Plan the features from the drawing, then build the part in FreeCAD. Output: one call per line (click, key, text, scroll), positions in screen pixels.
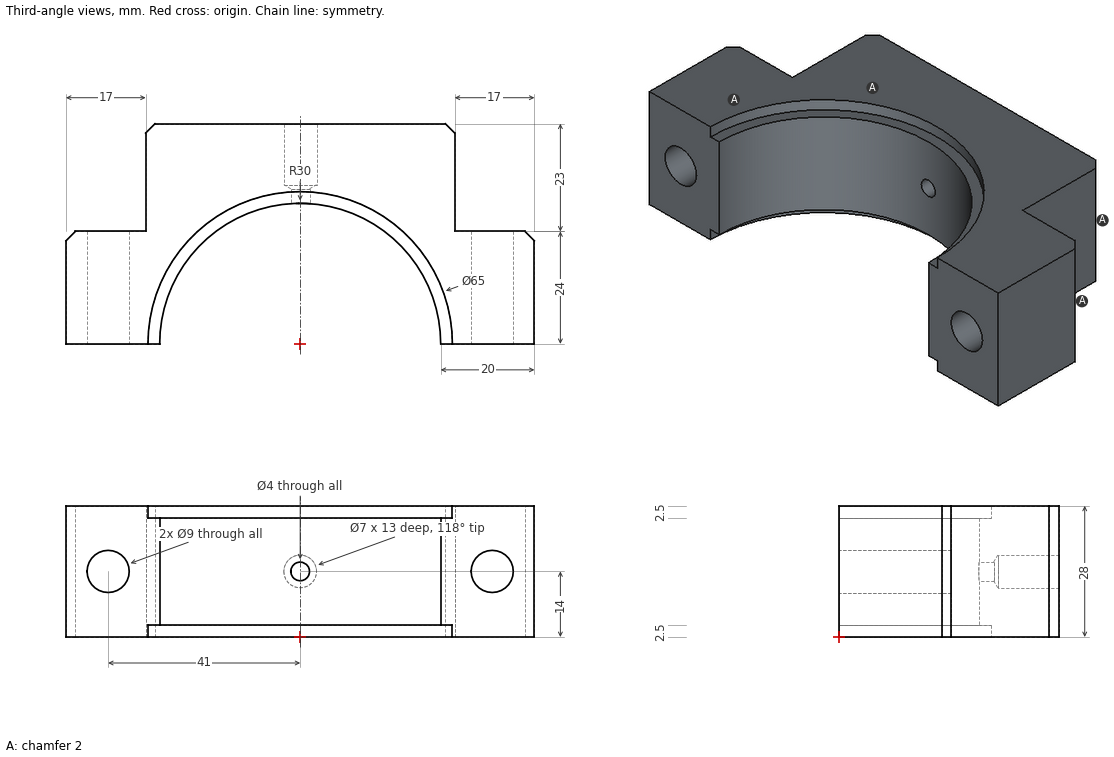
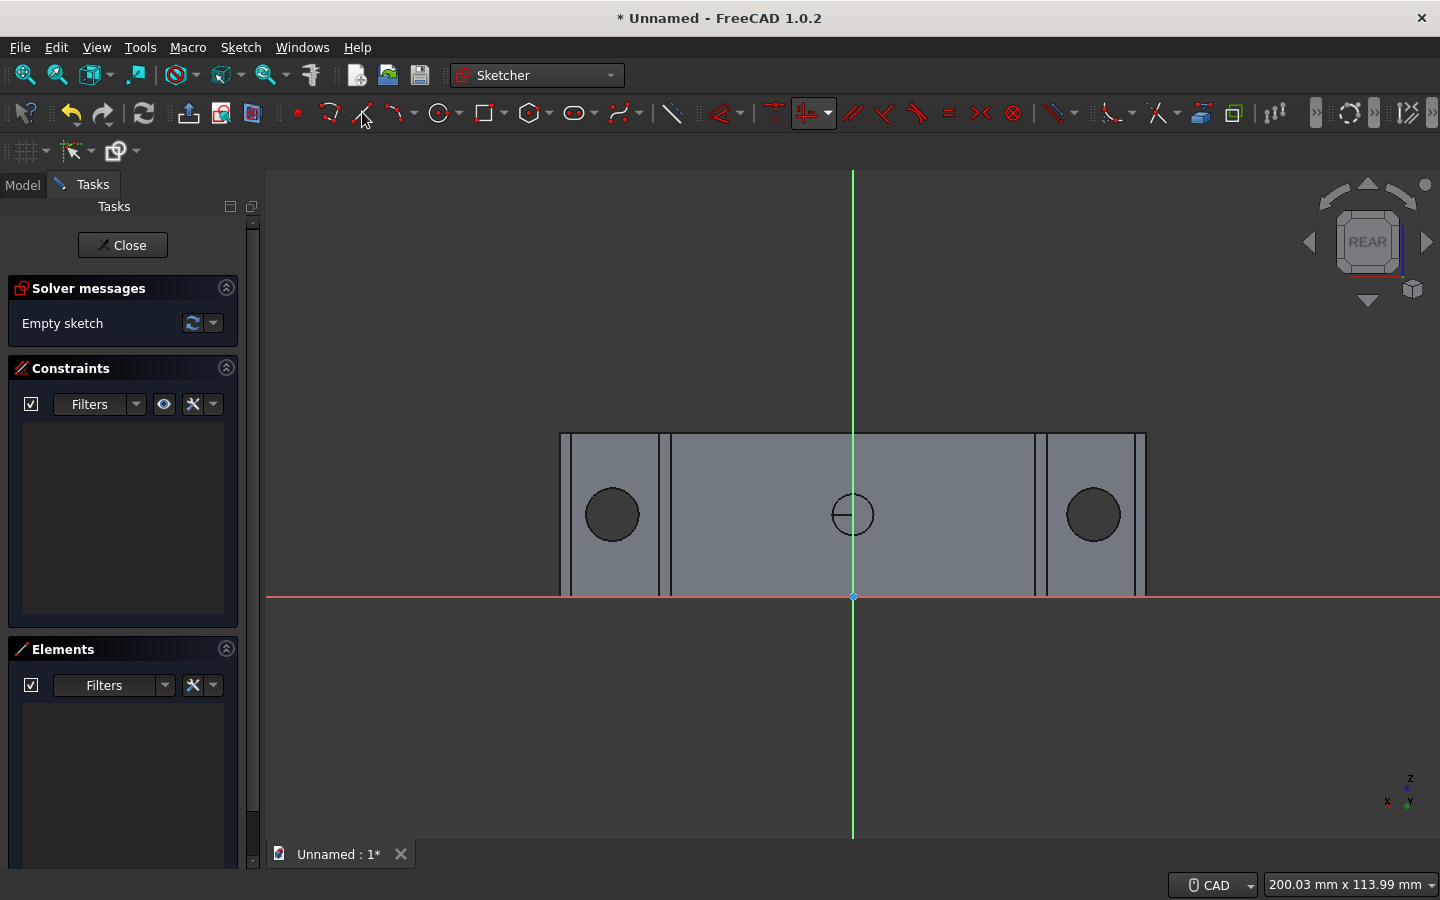
scroll(857, 515, up, 15)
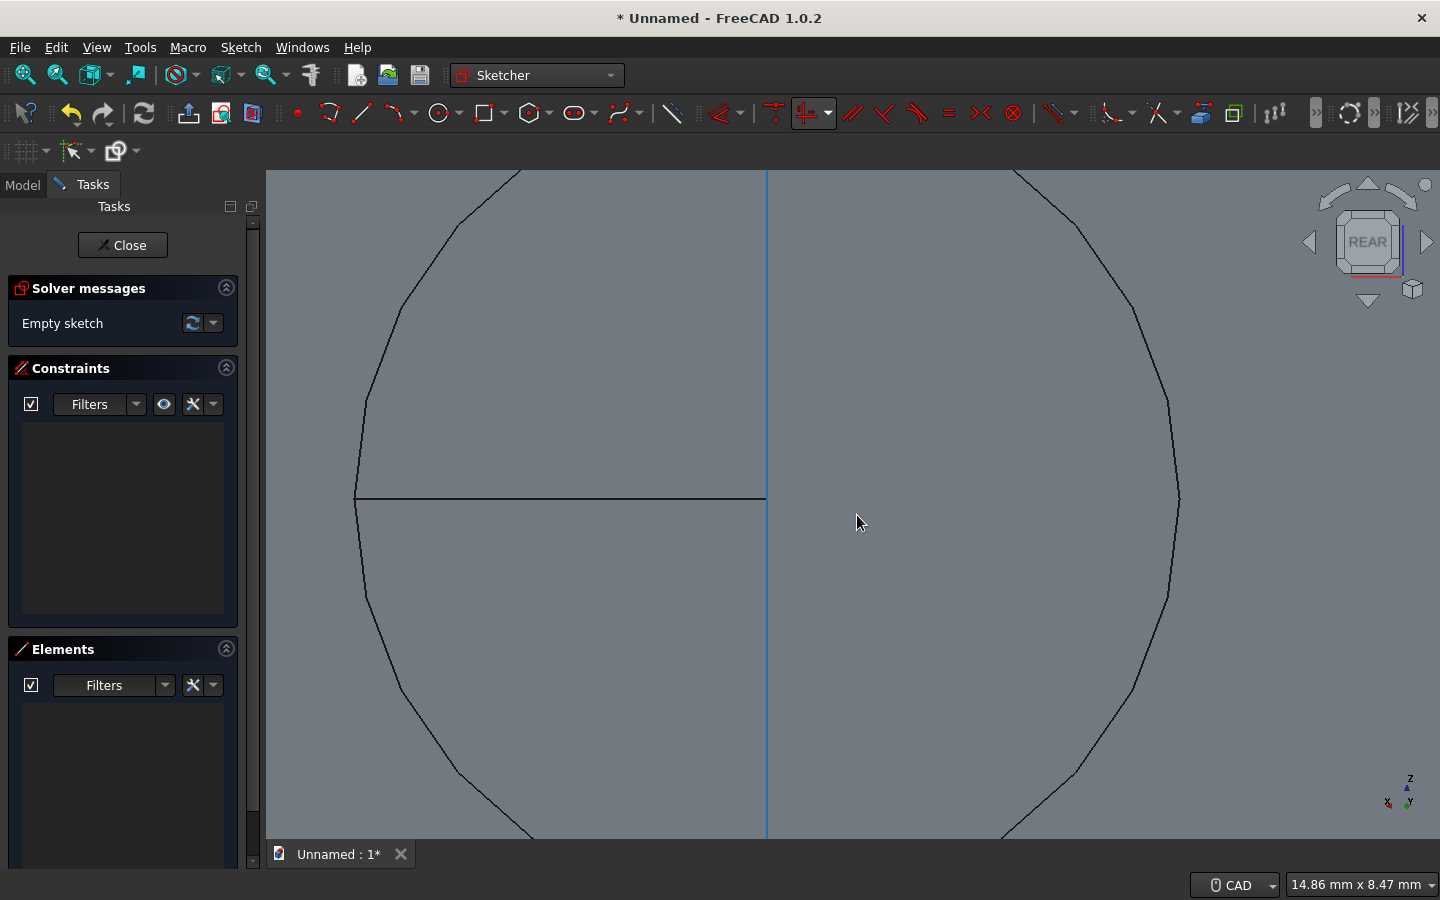
click(440, 114)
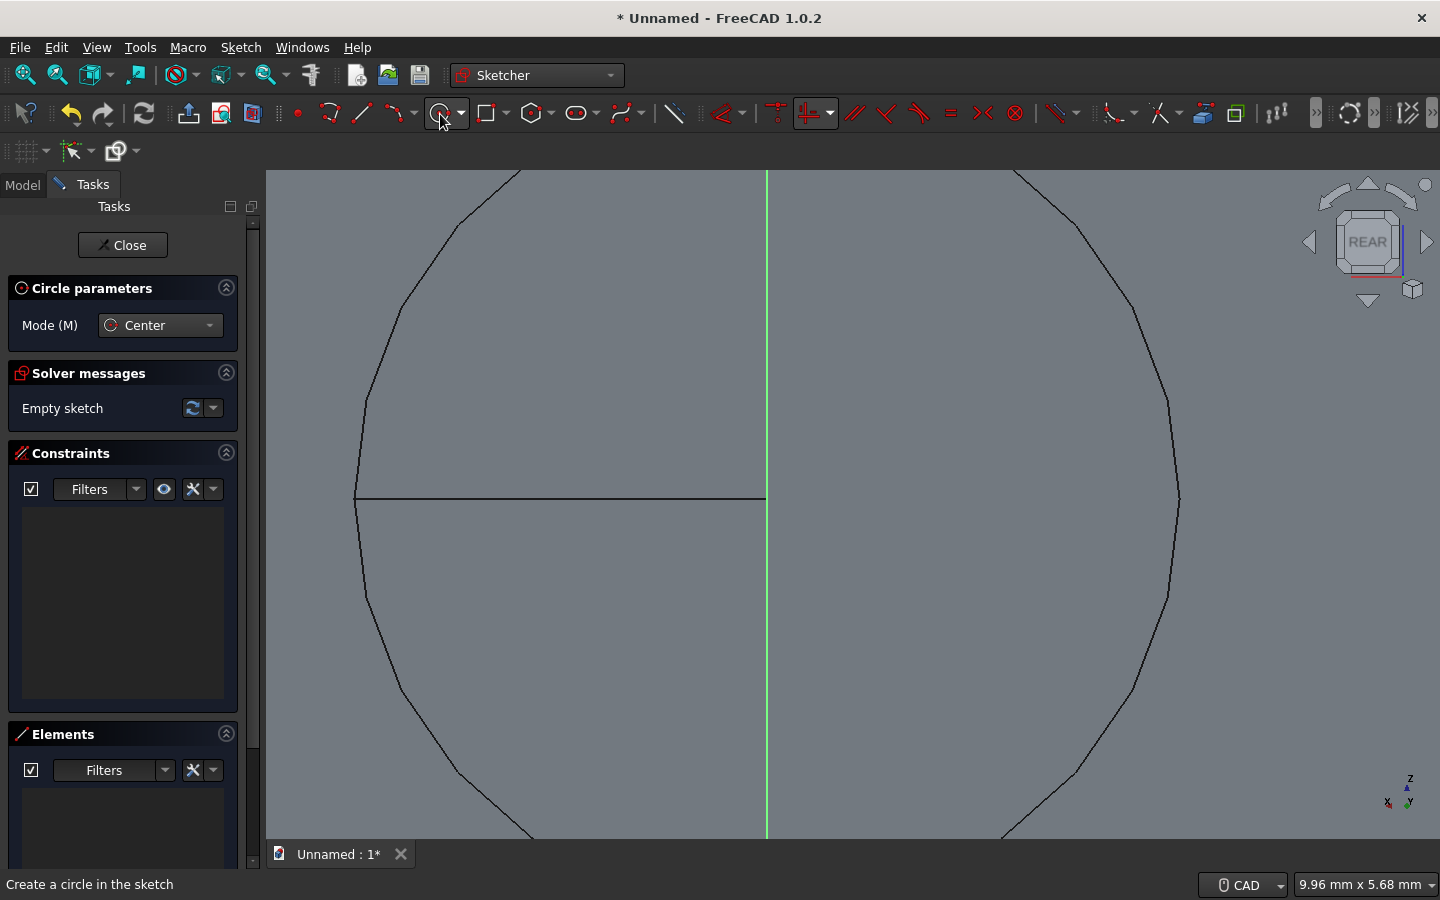
click(767, 499)
click(934, 332)
key(Escape)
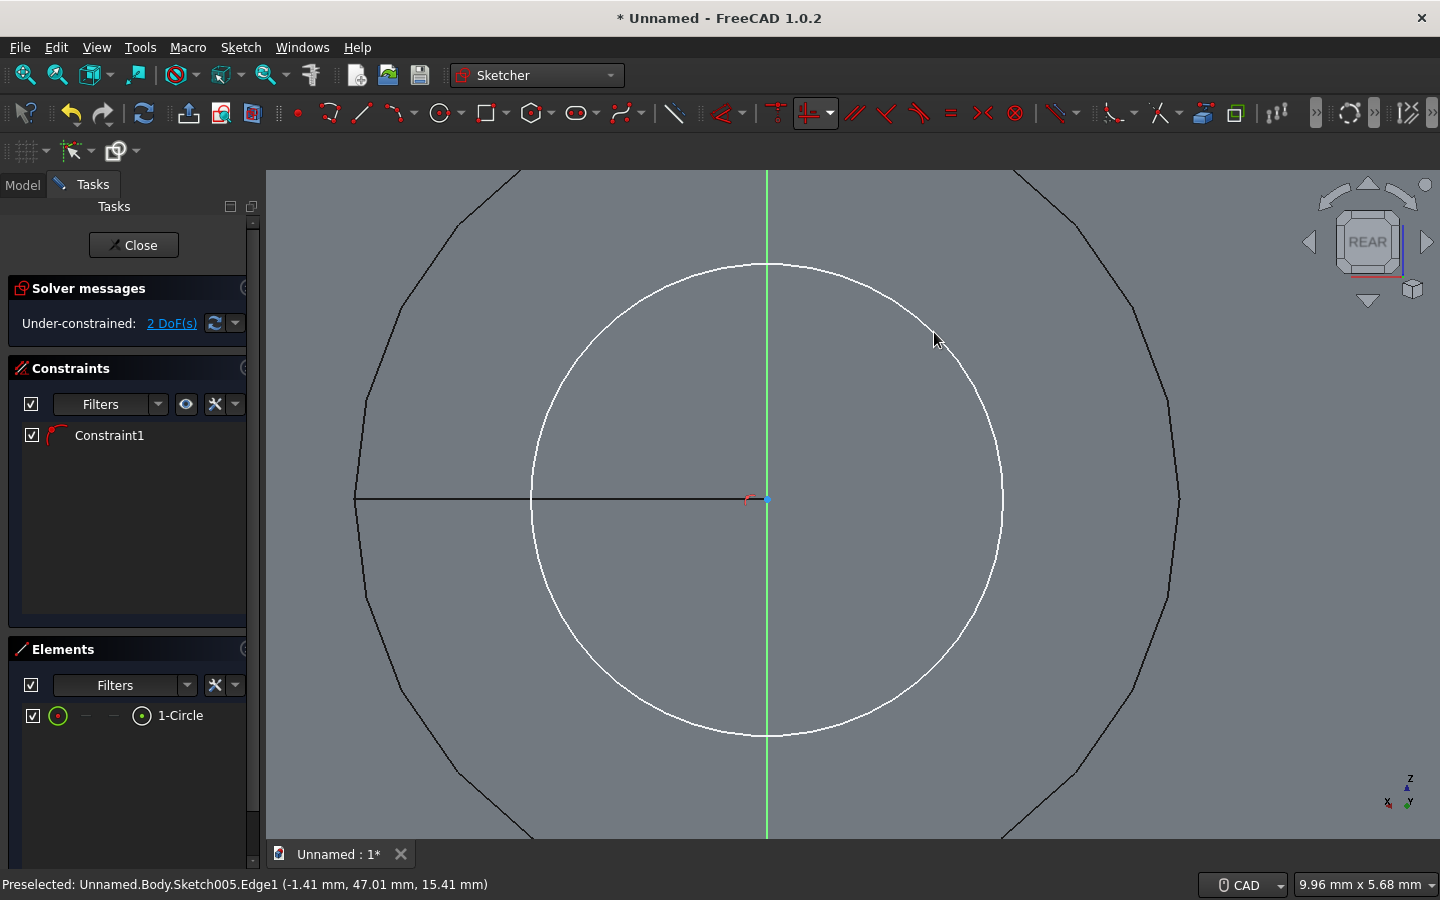
click(722, 114)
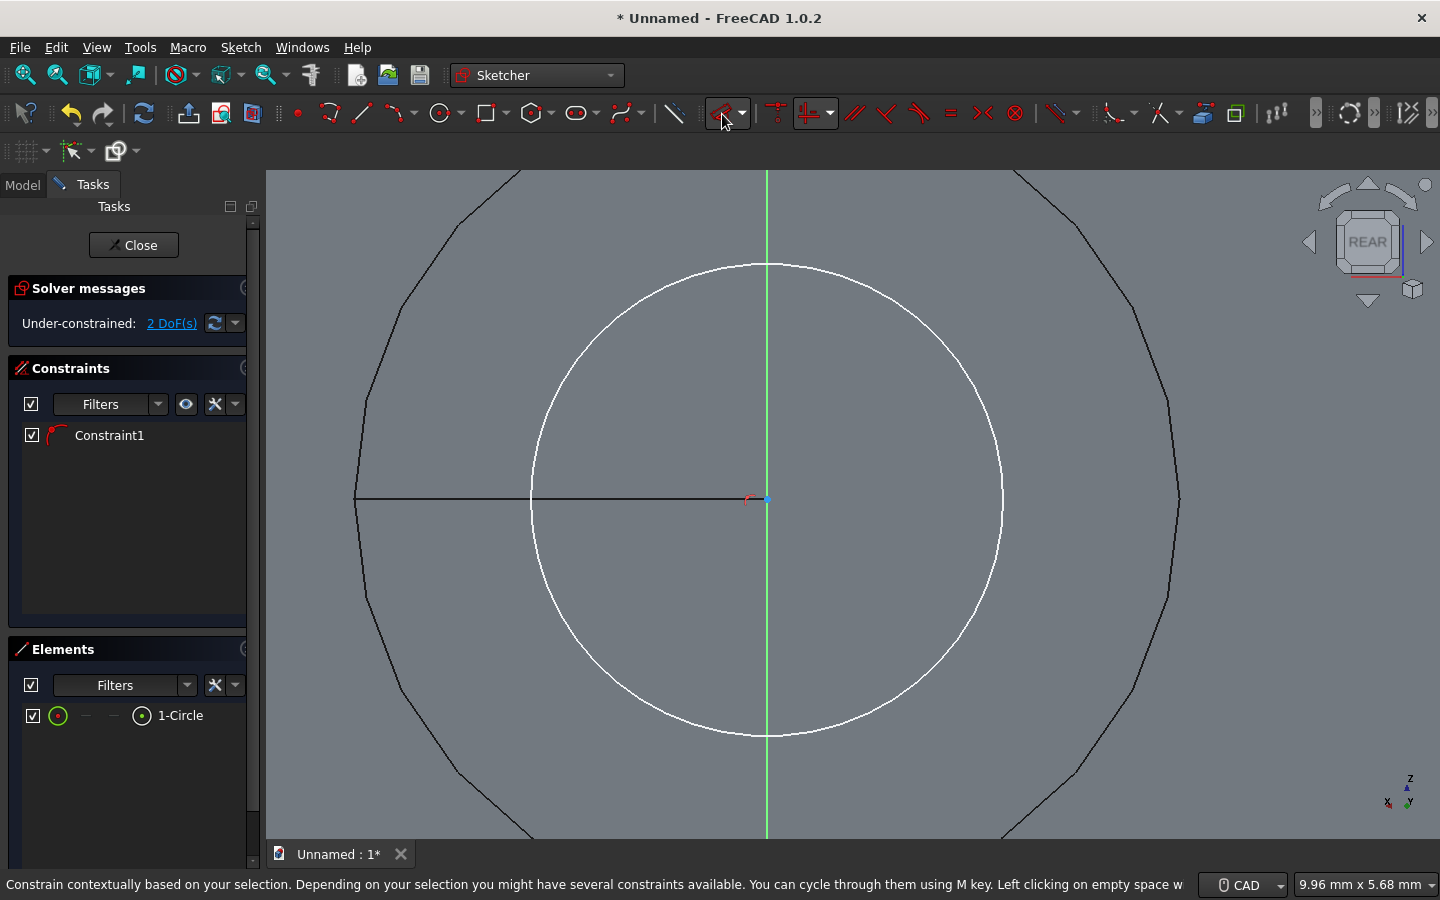
click(934, 333)
click(957, 310)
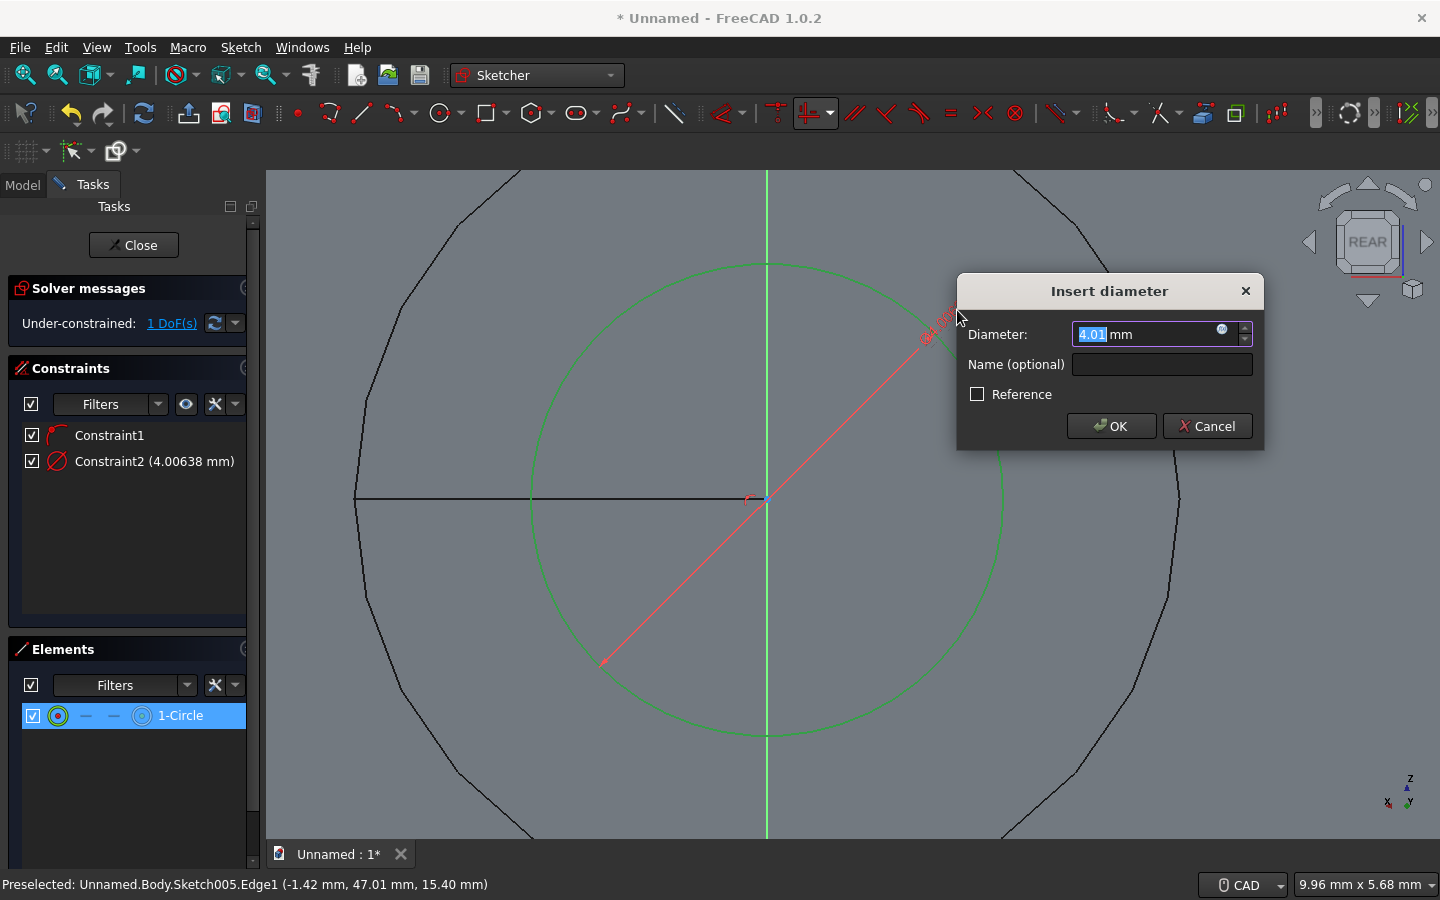
text(4)
key(Return)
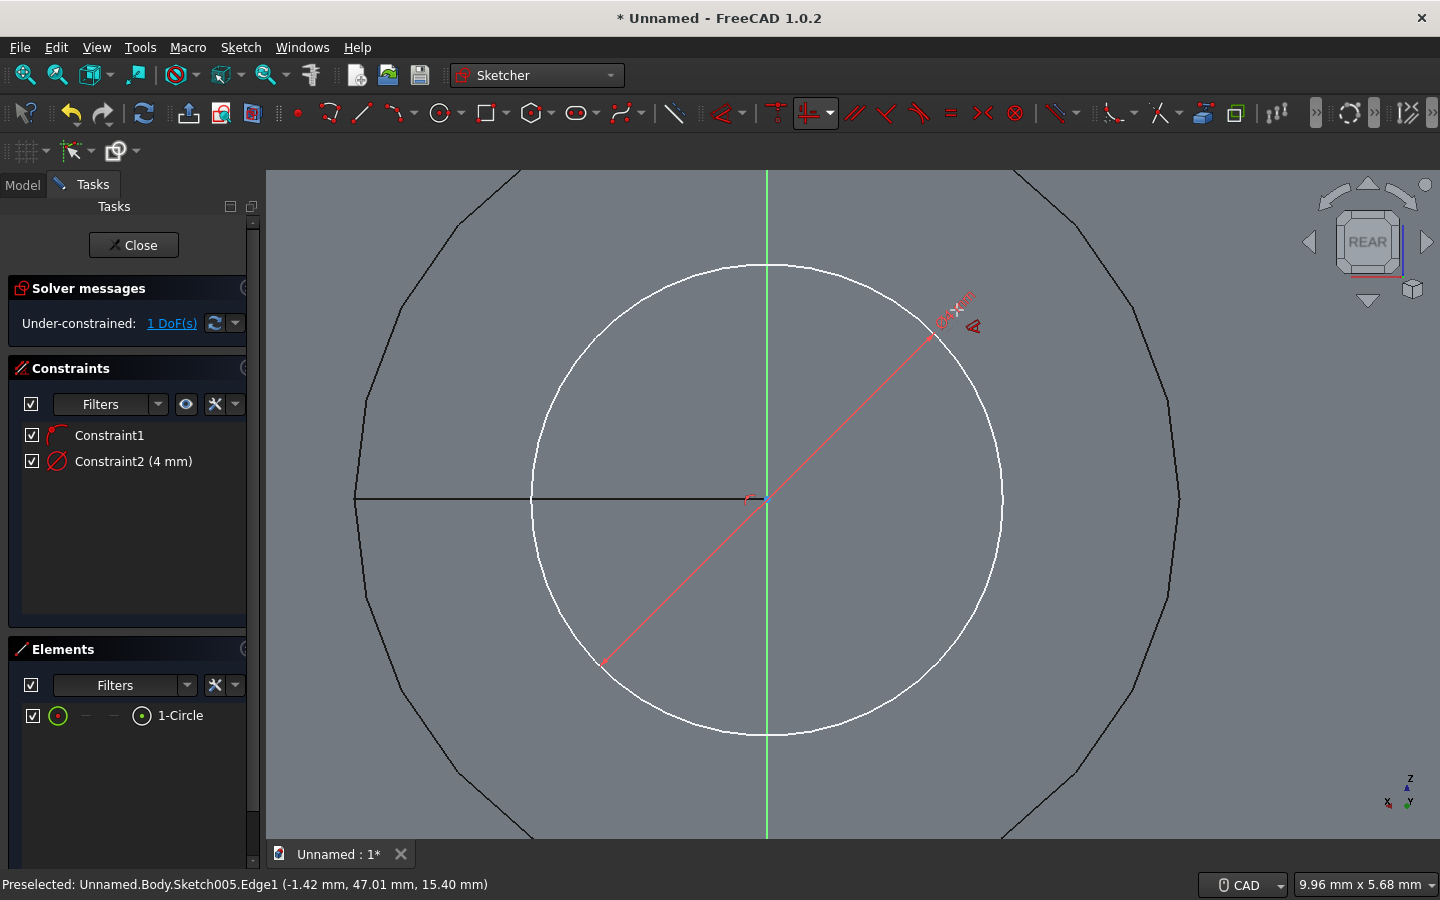
click(767, 500)
click(801, 656)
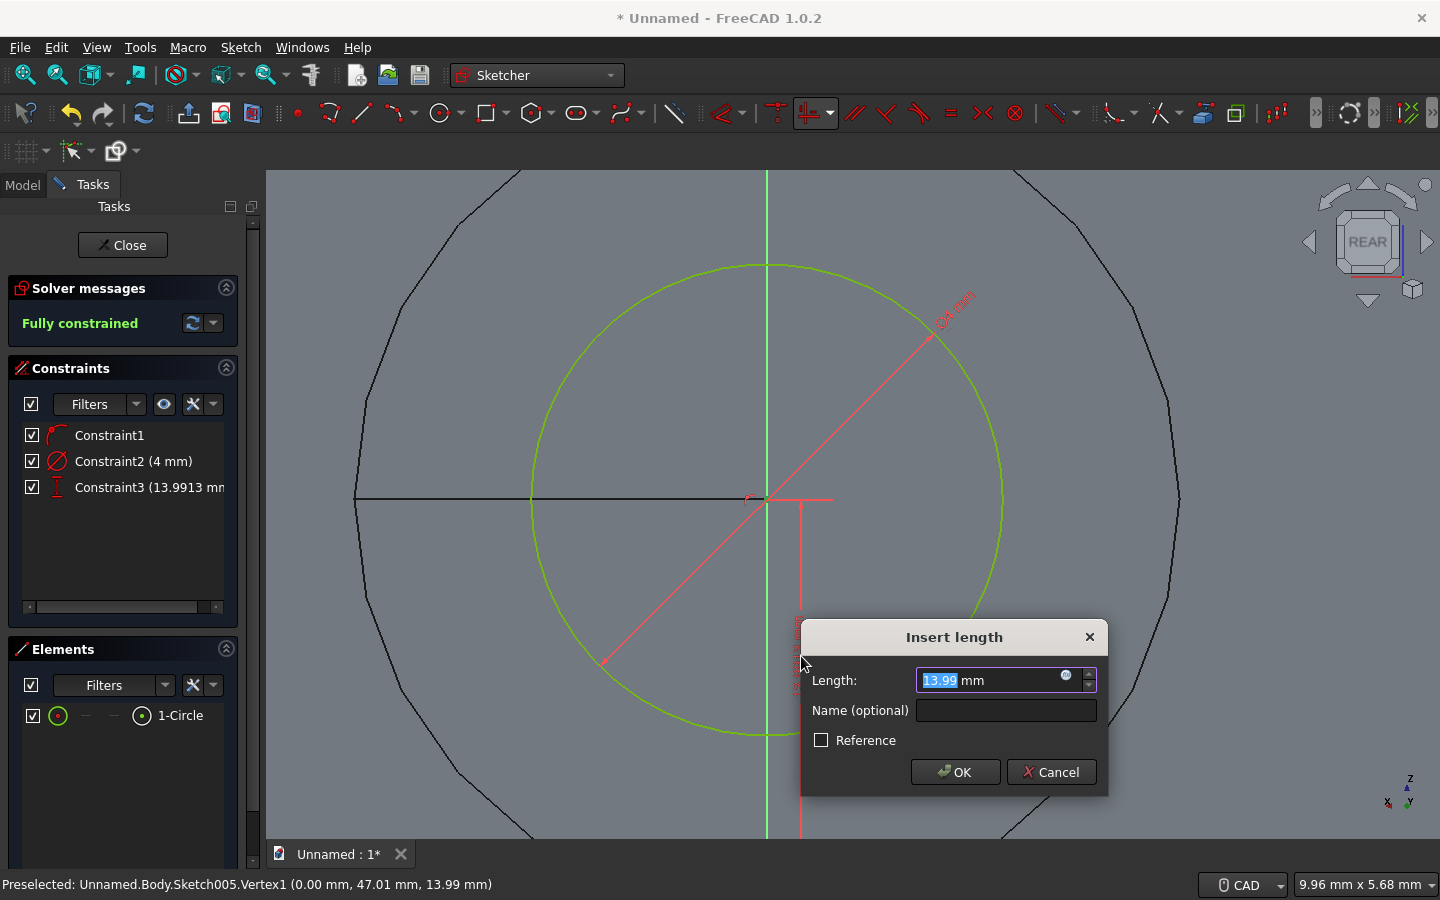
text(14)
key(Return)
key(Escape)